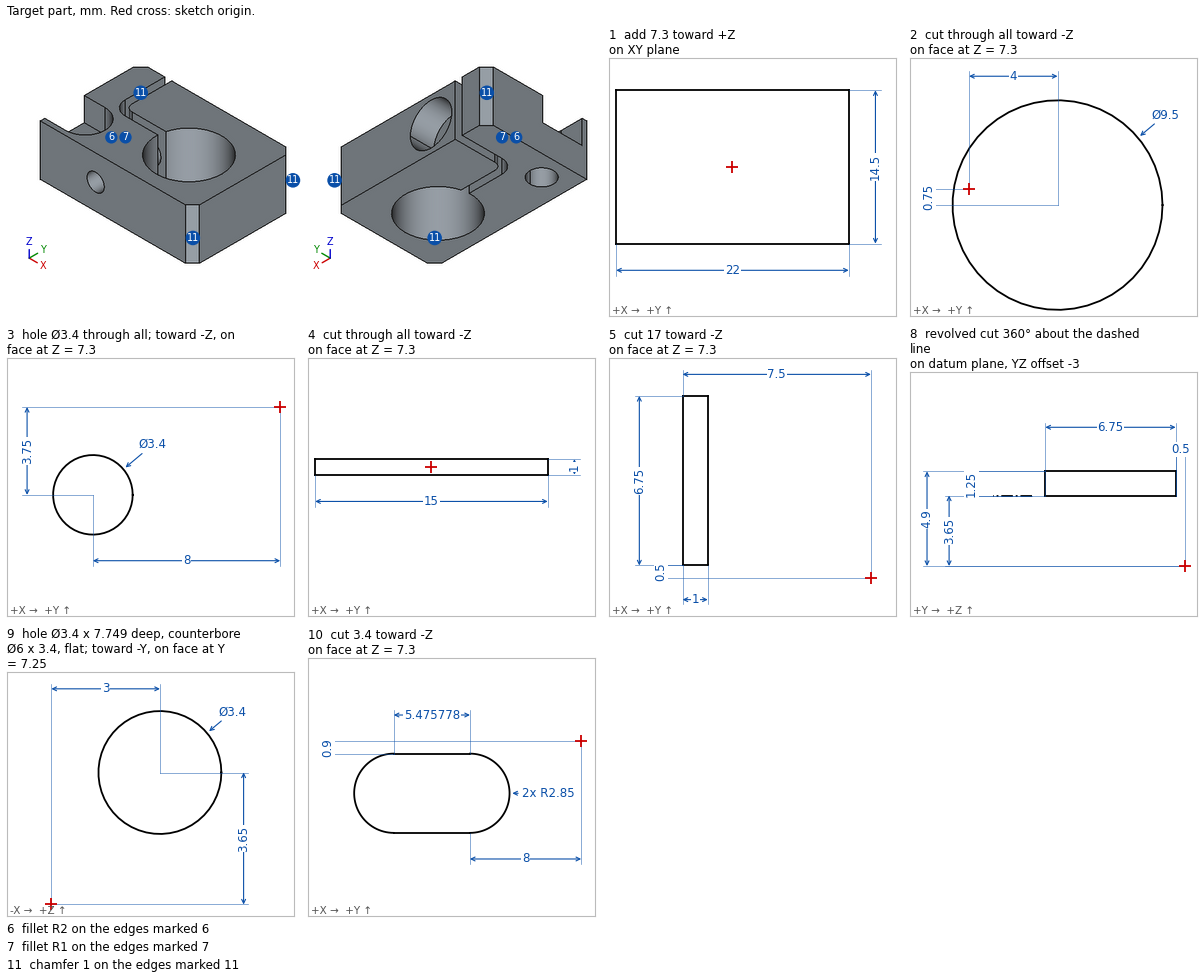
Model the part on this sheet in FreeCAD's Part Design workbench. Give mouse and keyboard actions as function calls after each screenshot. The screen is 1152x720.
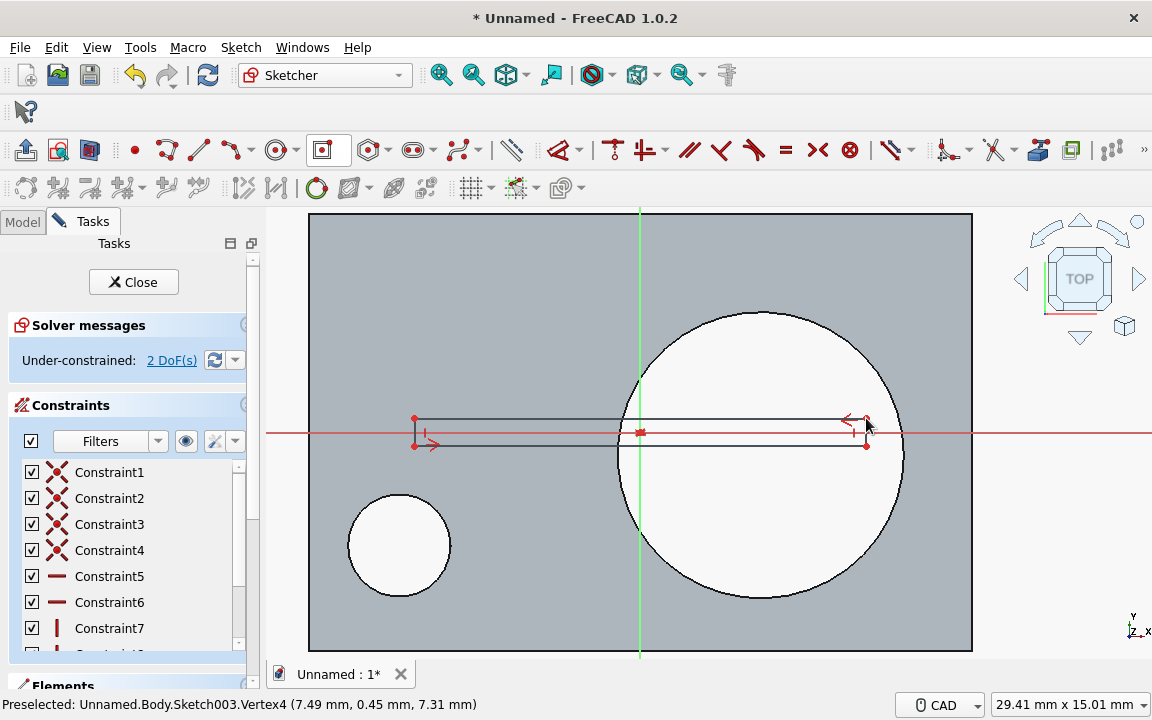
click(558, 150)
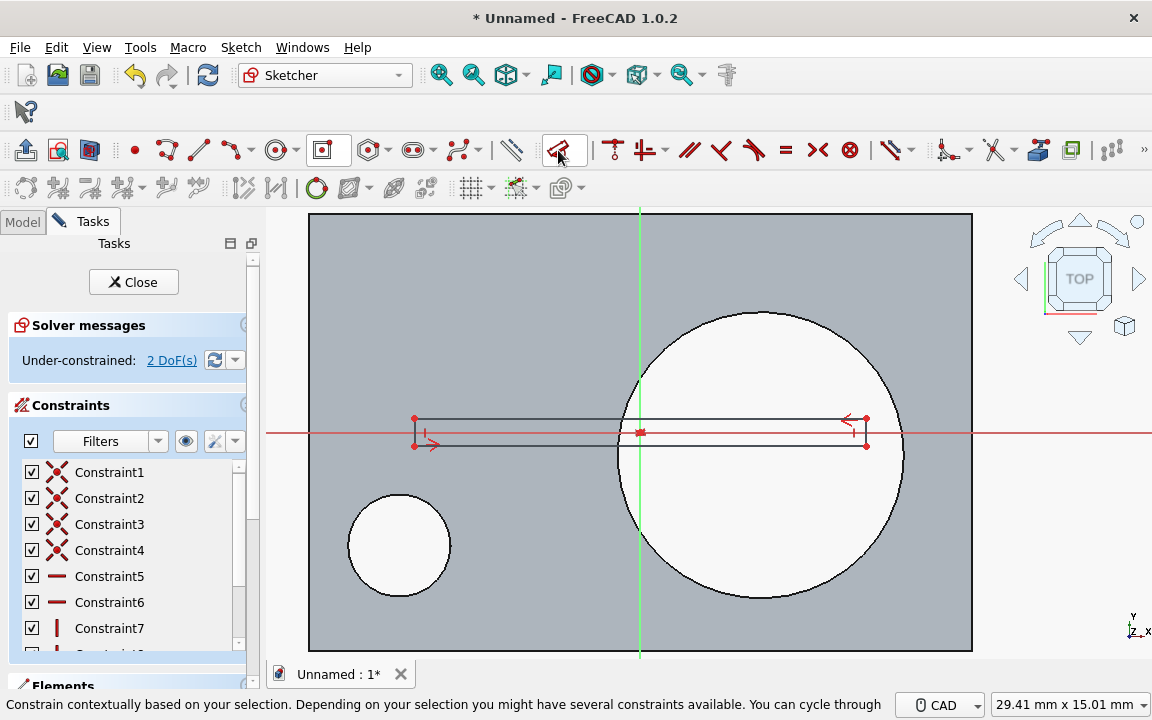
scroll(866, 435, up, 2)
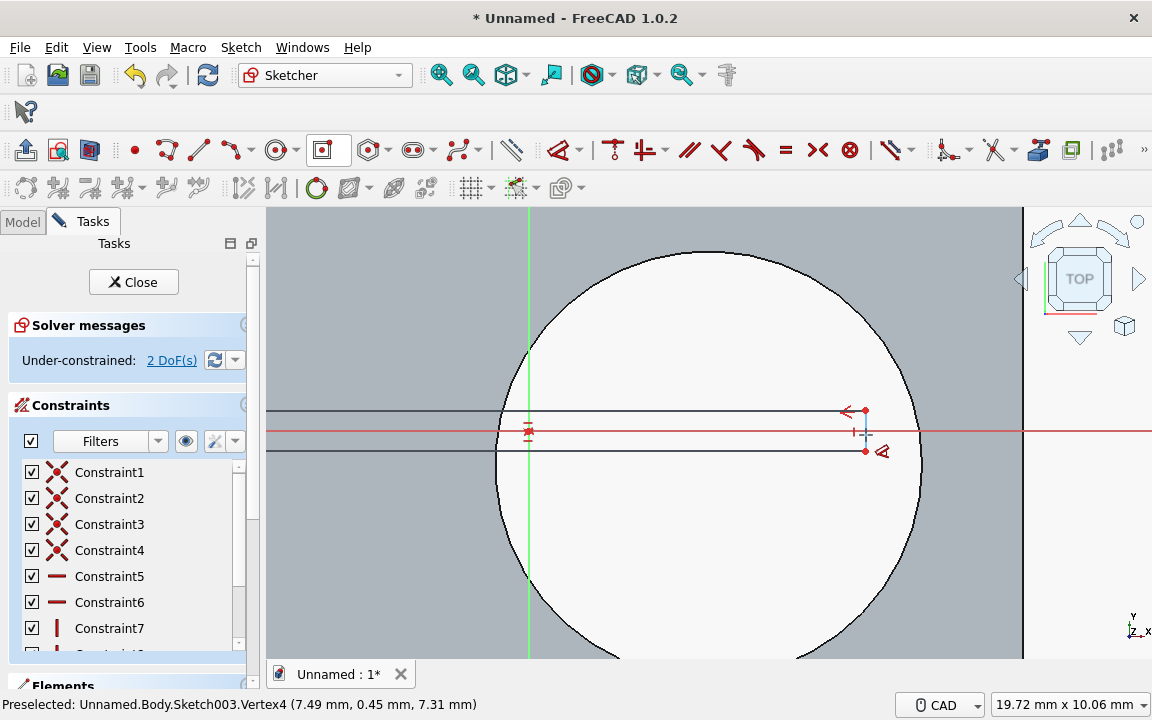
click(866, 435)
click(900, 417)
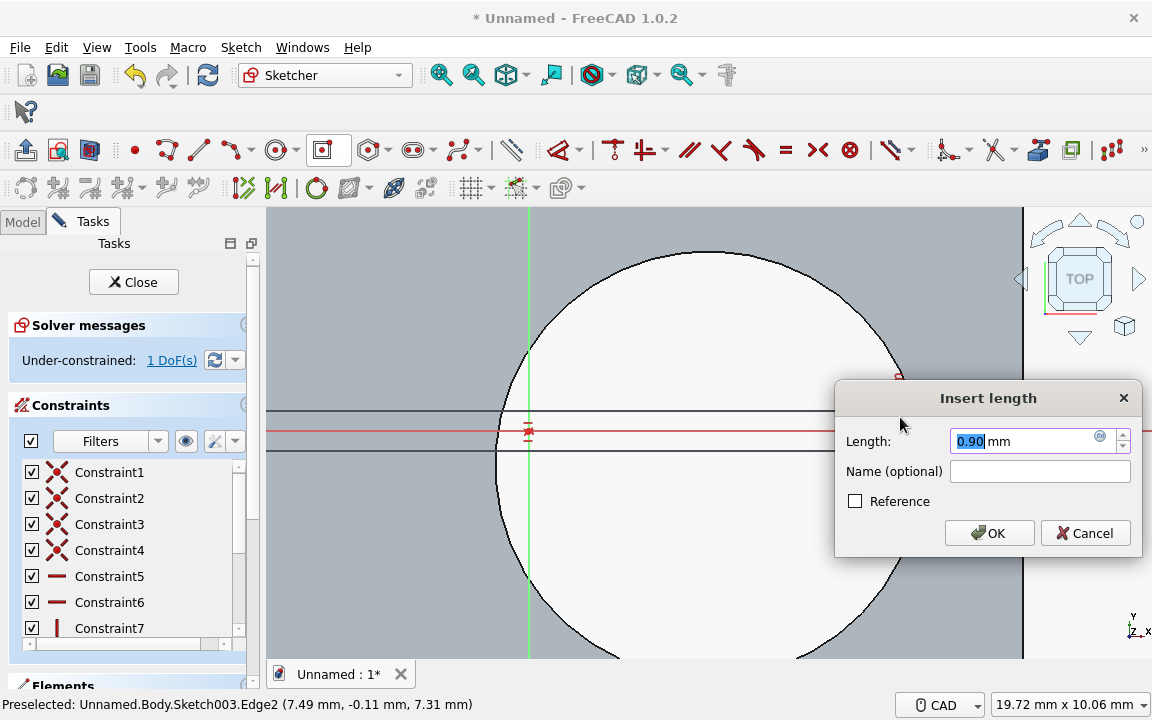
text(1)
key(Return)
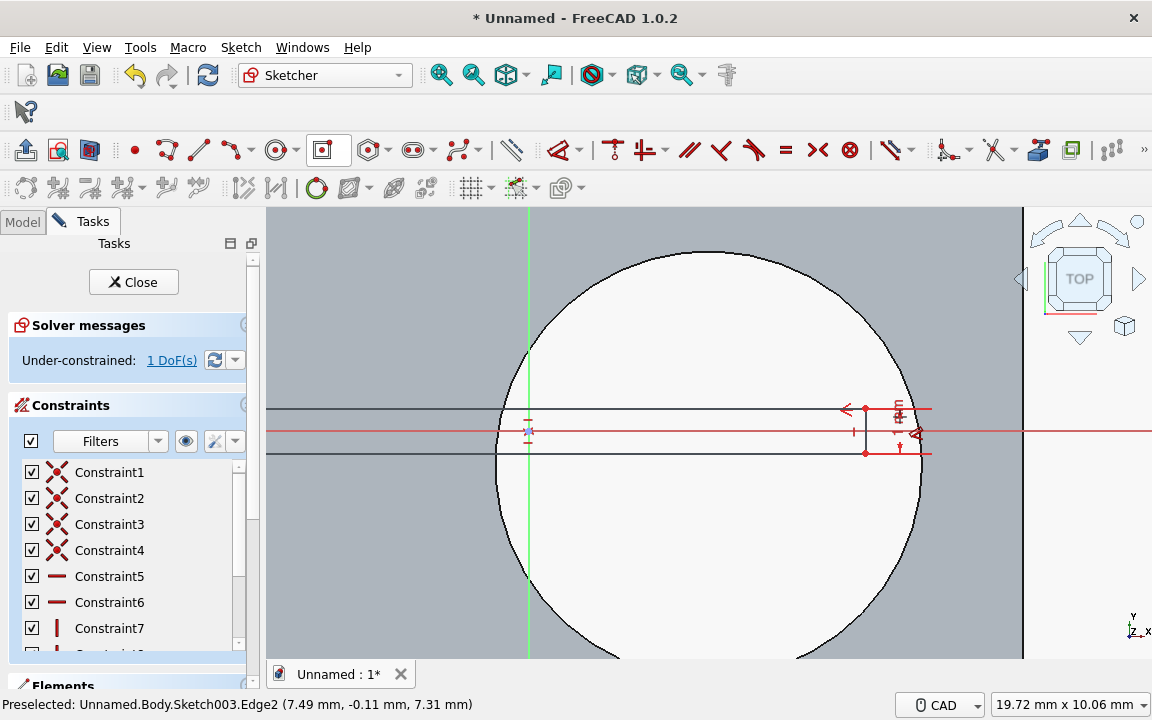
click(394, 454)
click(580, 488)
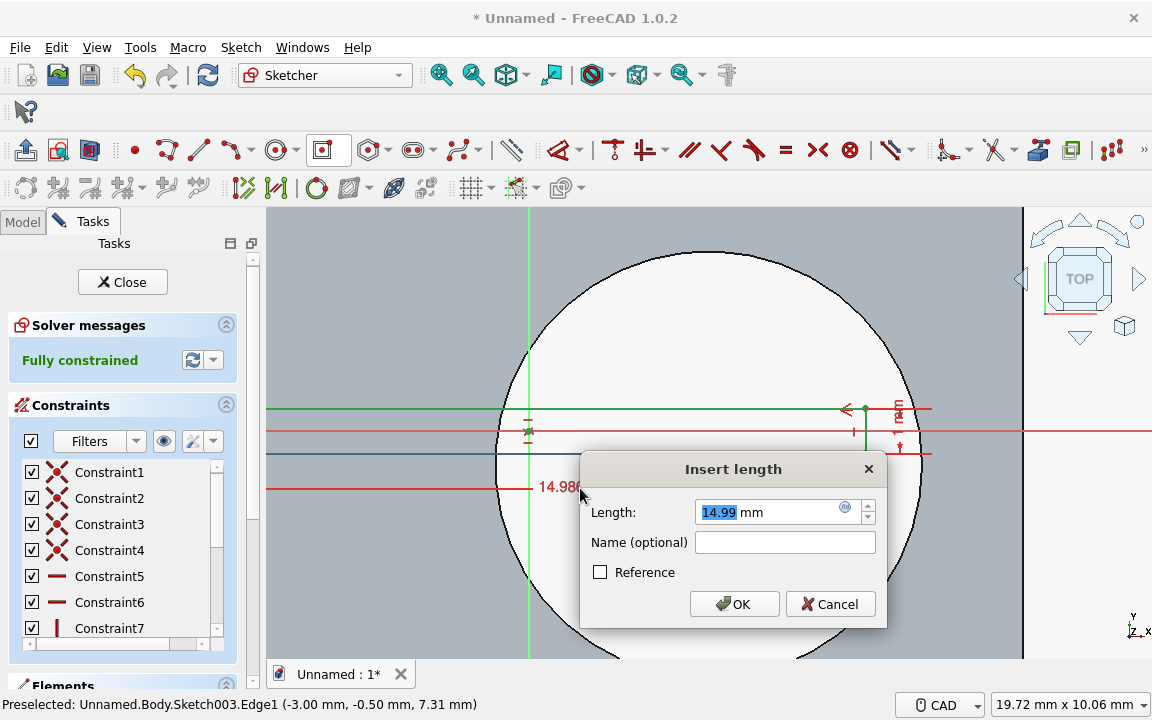
text(15)
key(Return)
key(Escape)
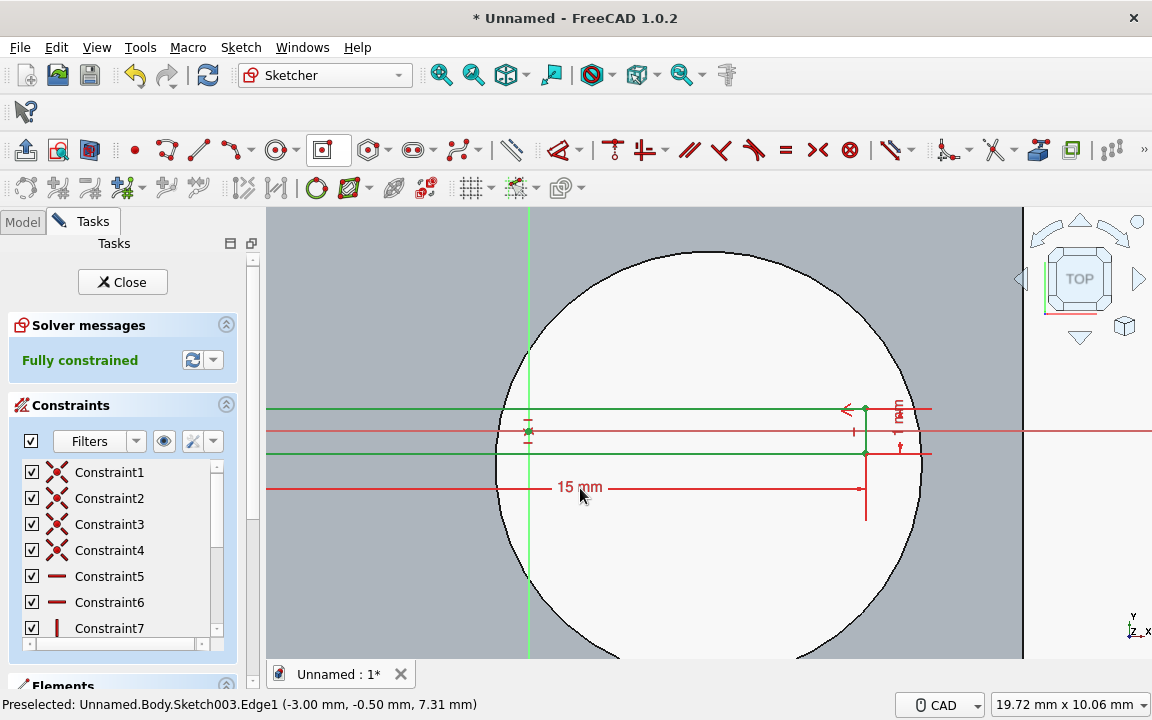
click(123, 282)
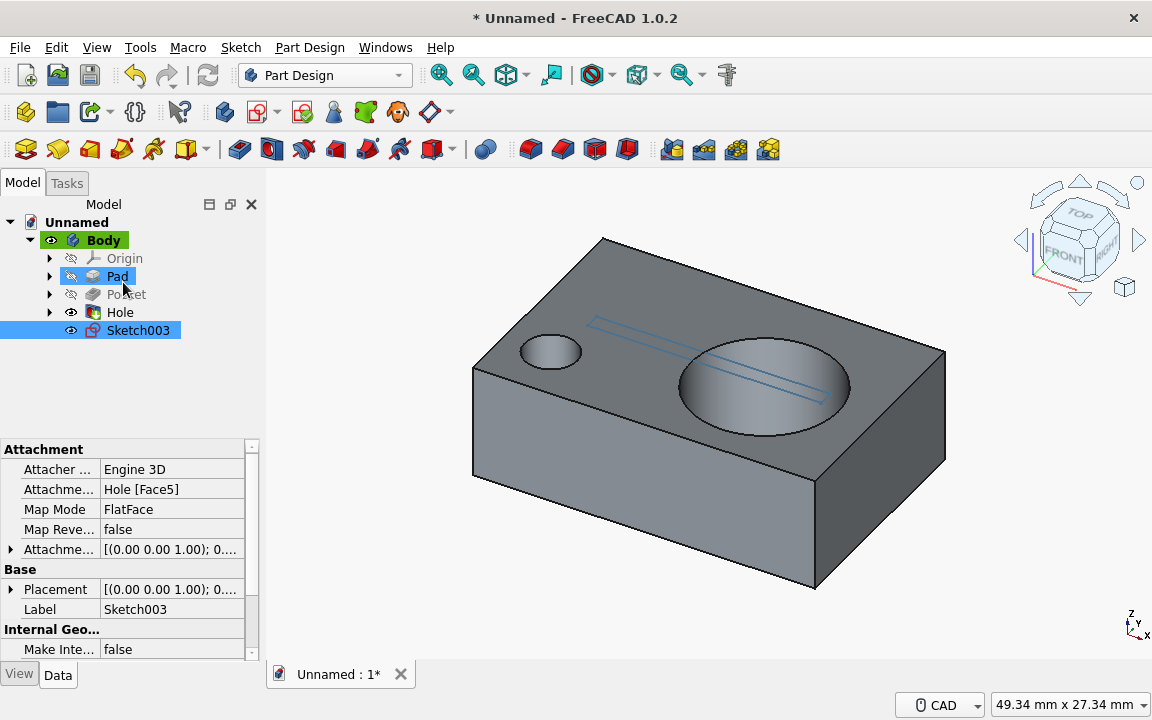
click(240, 150)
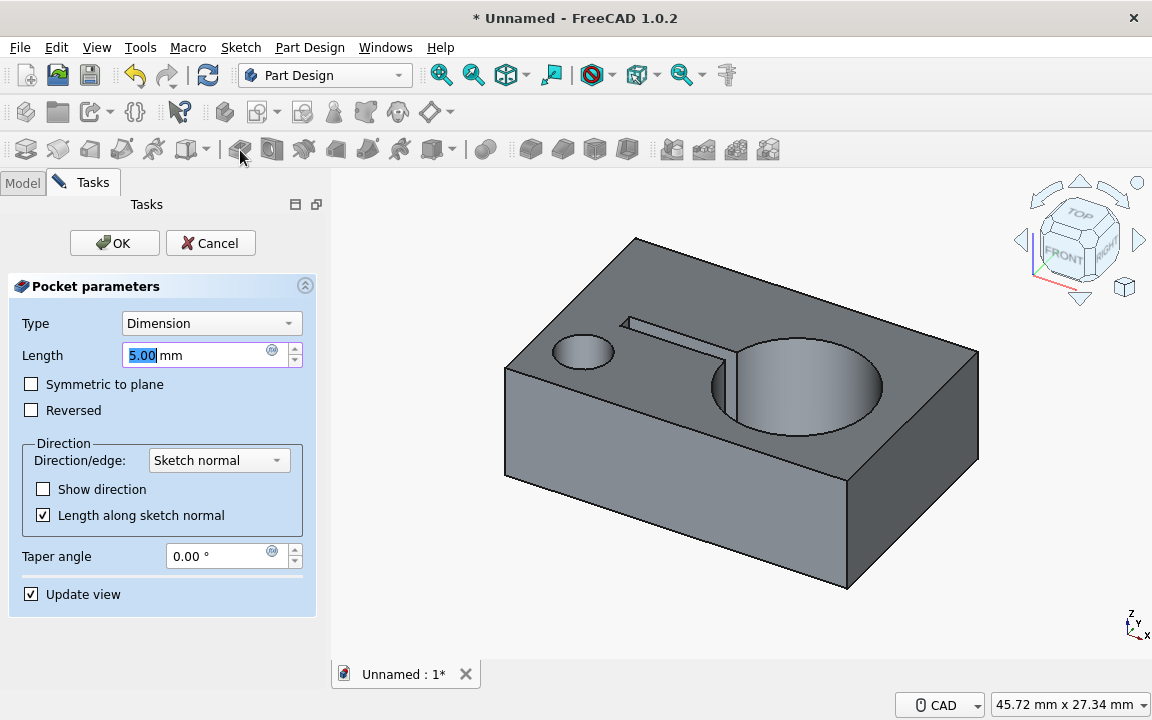
click(212, 324)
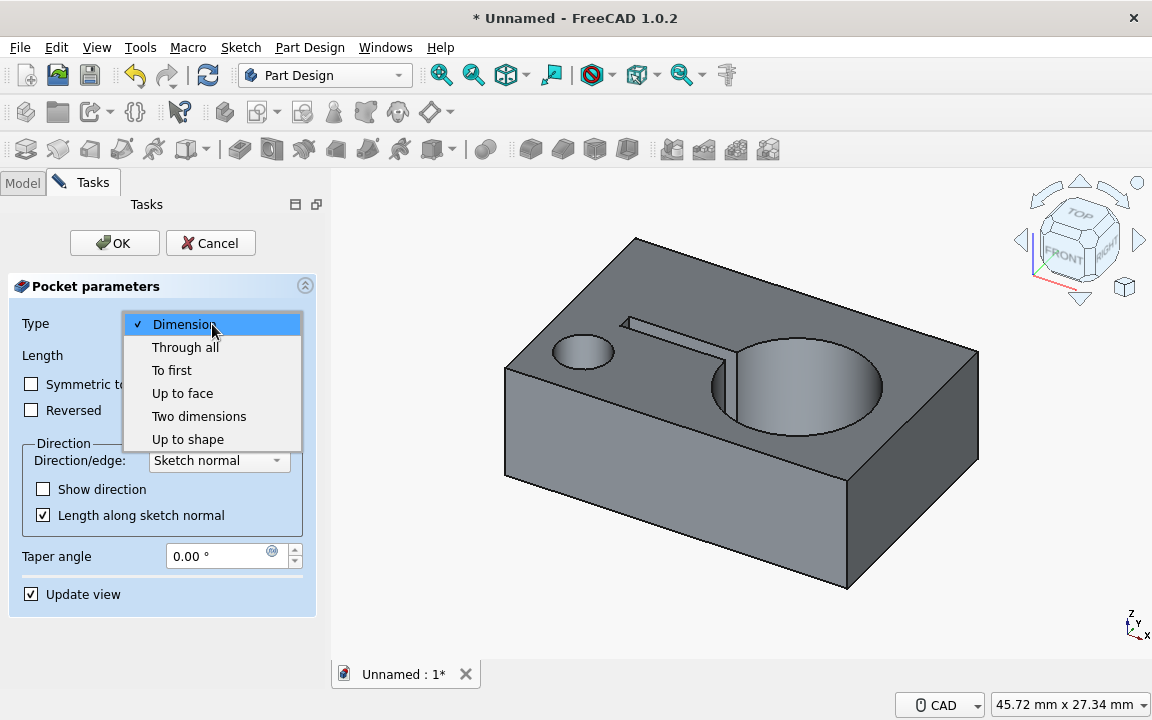
click(212, 348)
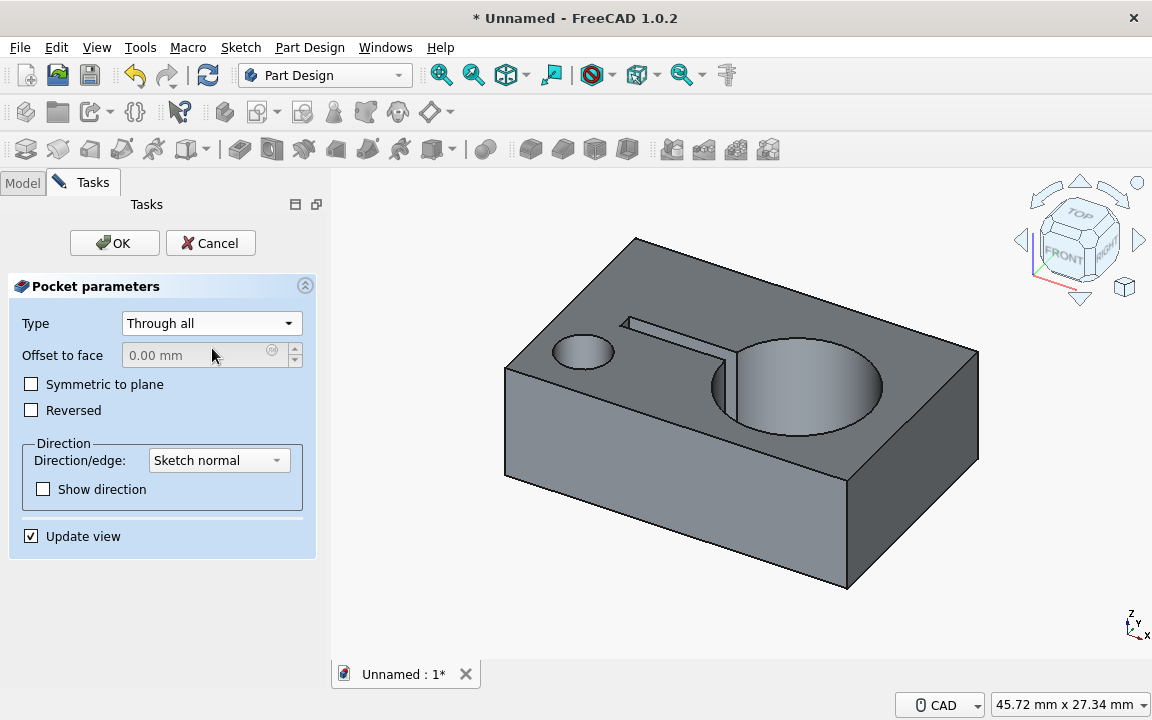
click(115, 243)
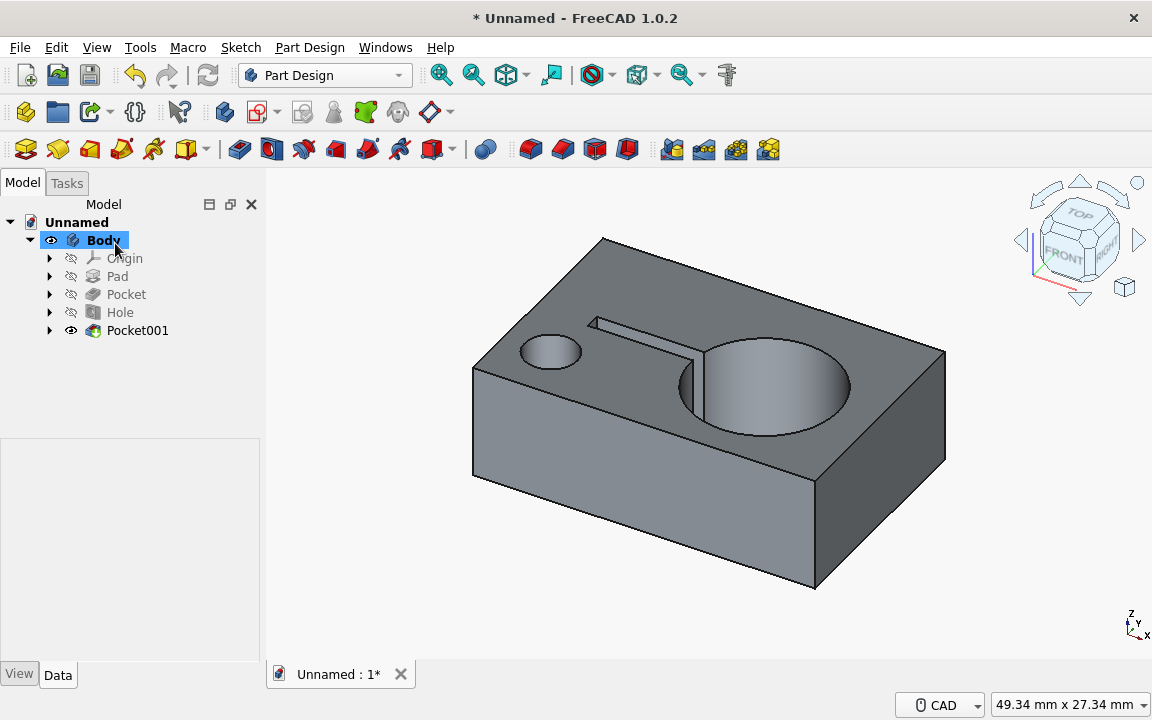
click(697, 306)